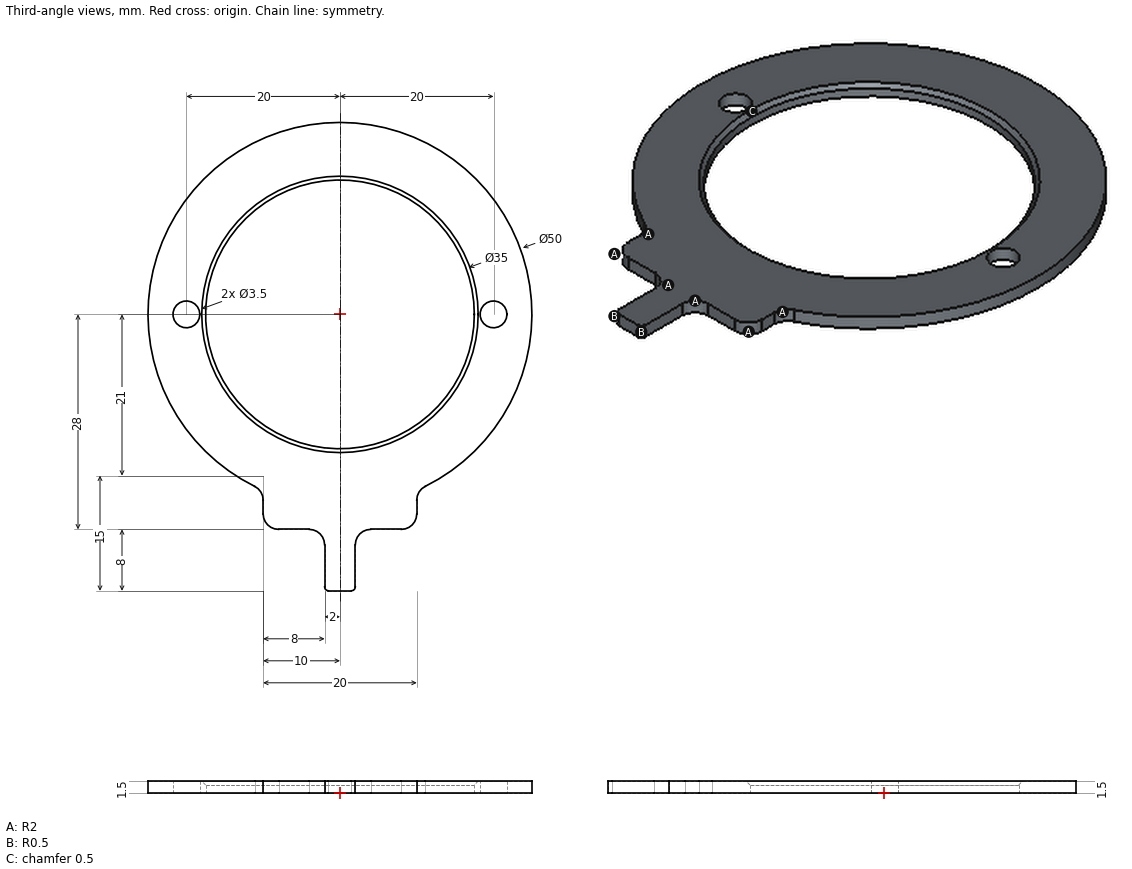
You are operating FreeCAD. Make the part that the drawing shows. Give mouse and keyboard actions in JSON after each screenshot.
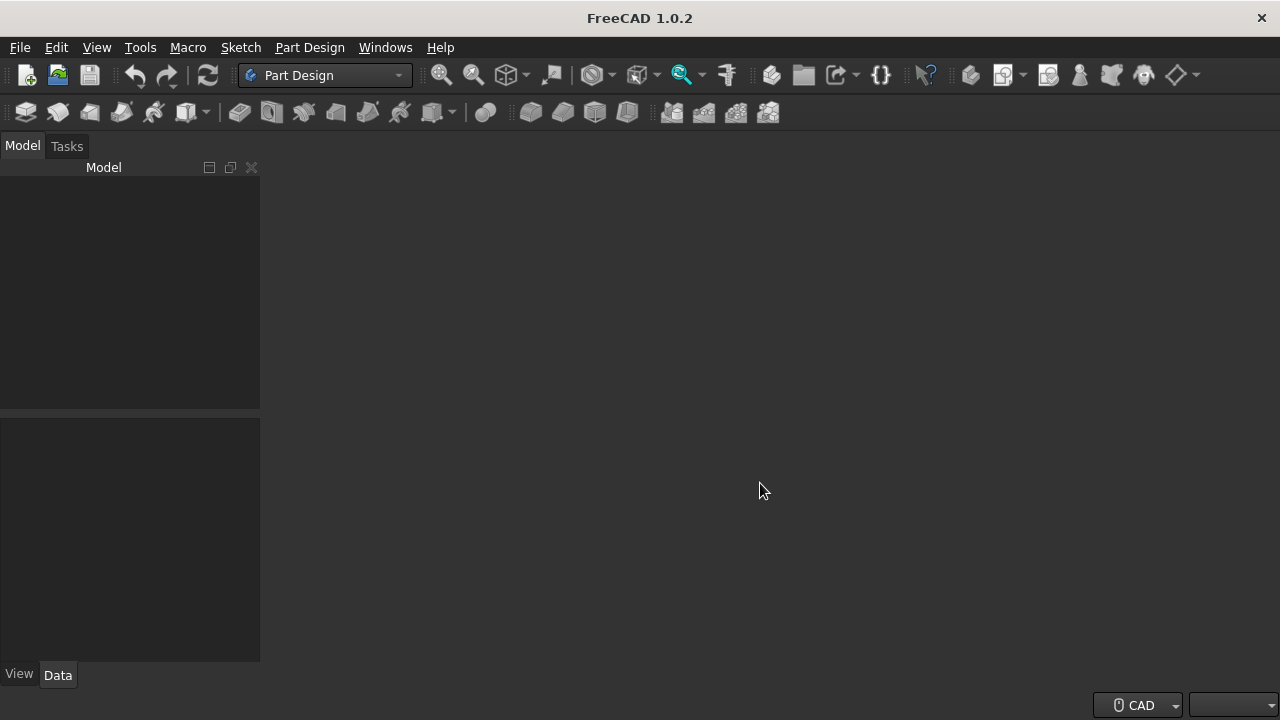
{"action": "left_click", "coordinate": [26, 76]}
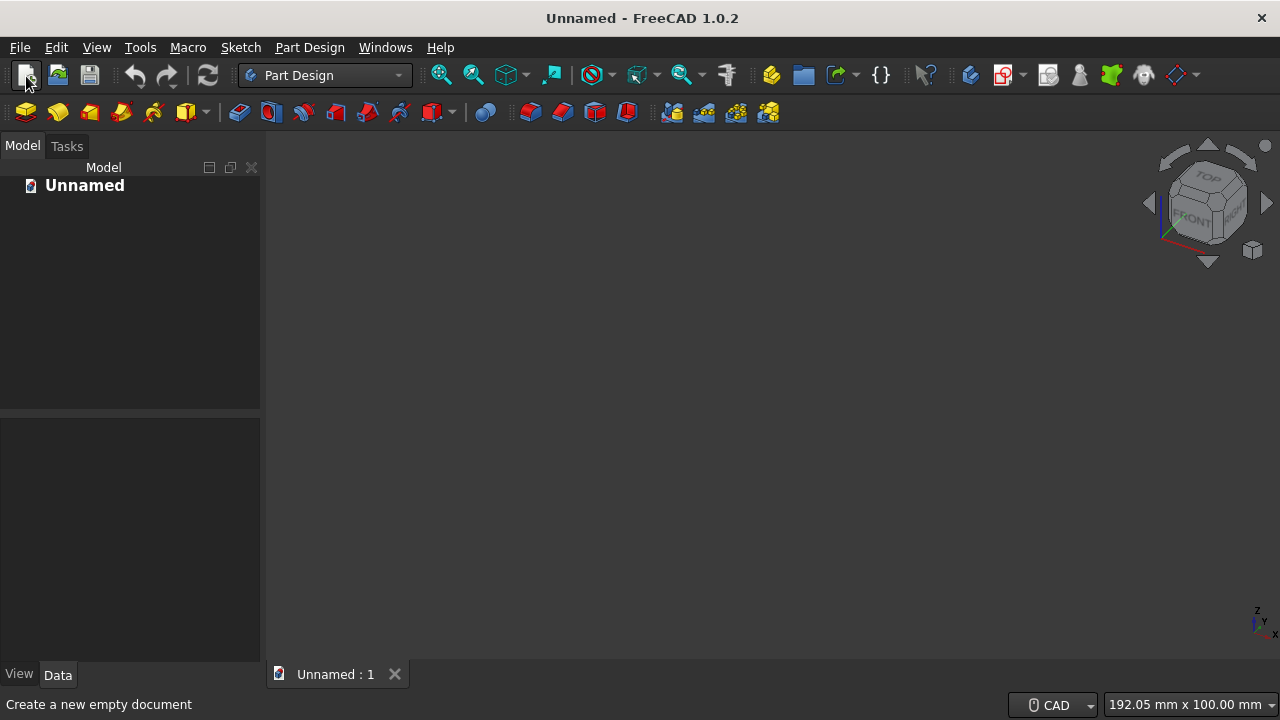
{"action": "left_click", "coordinate": [1004, 76]}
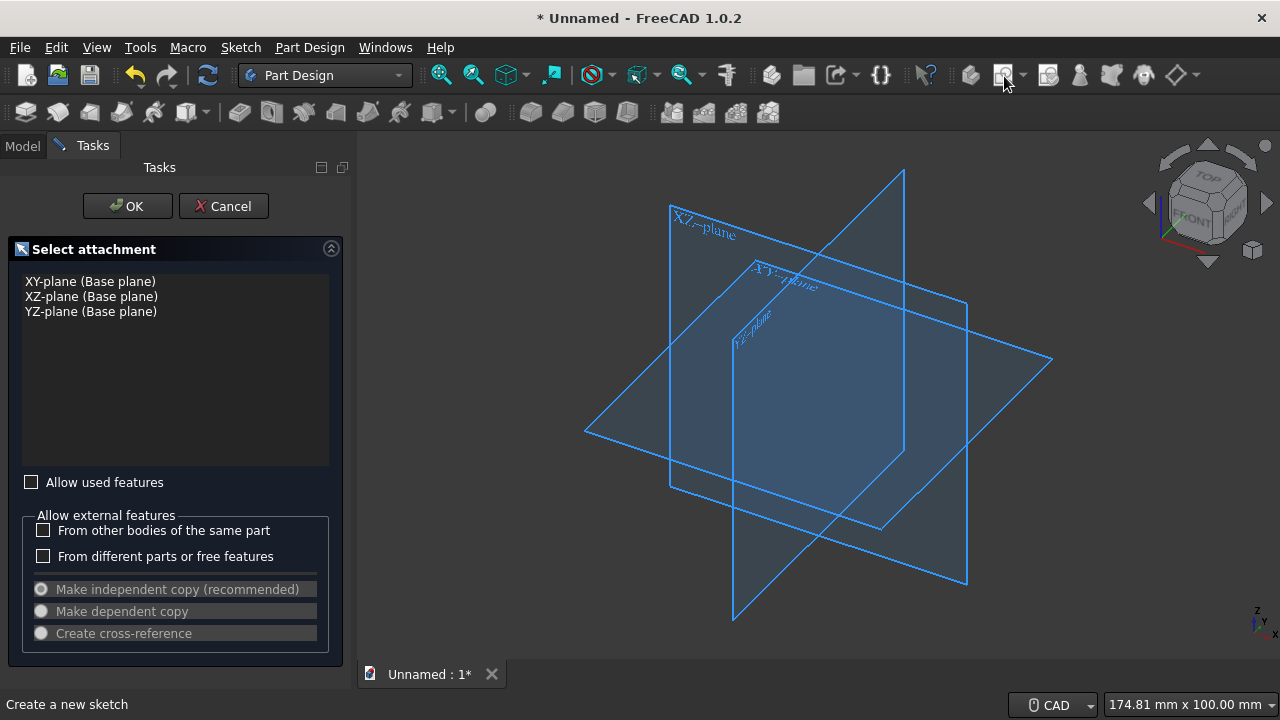
{"action": "left_click", "coordinate": [82, 282]}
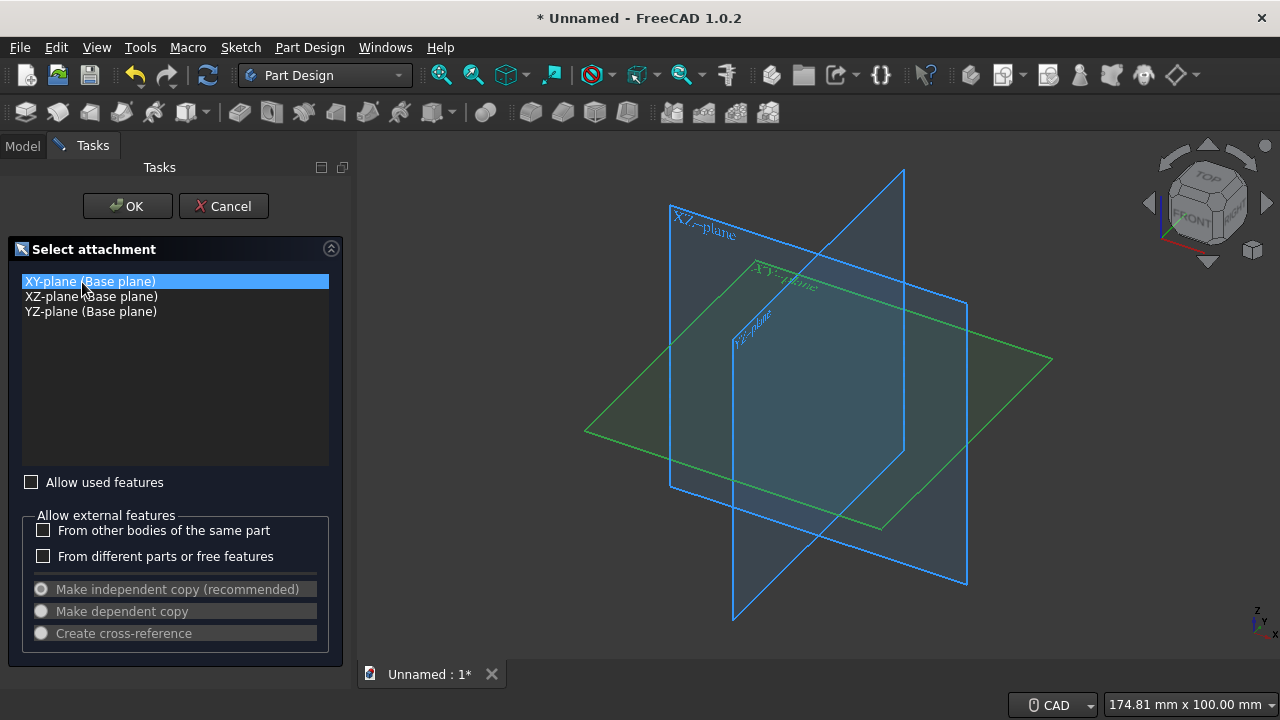
{"action": "left_click", "coordinate": [128, 206]}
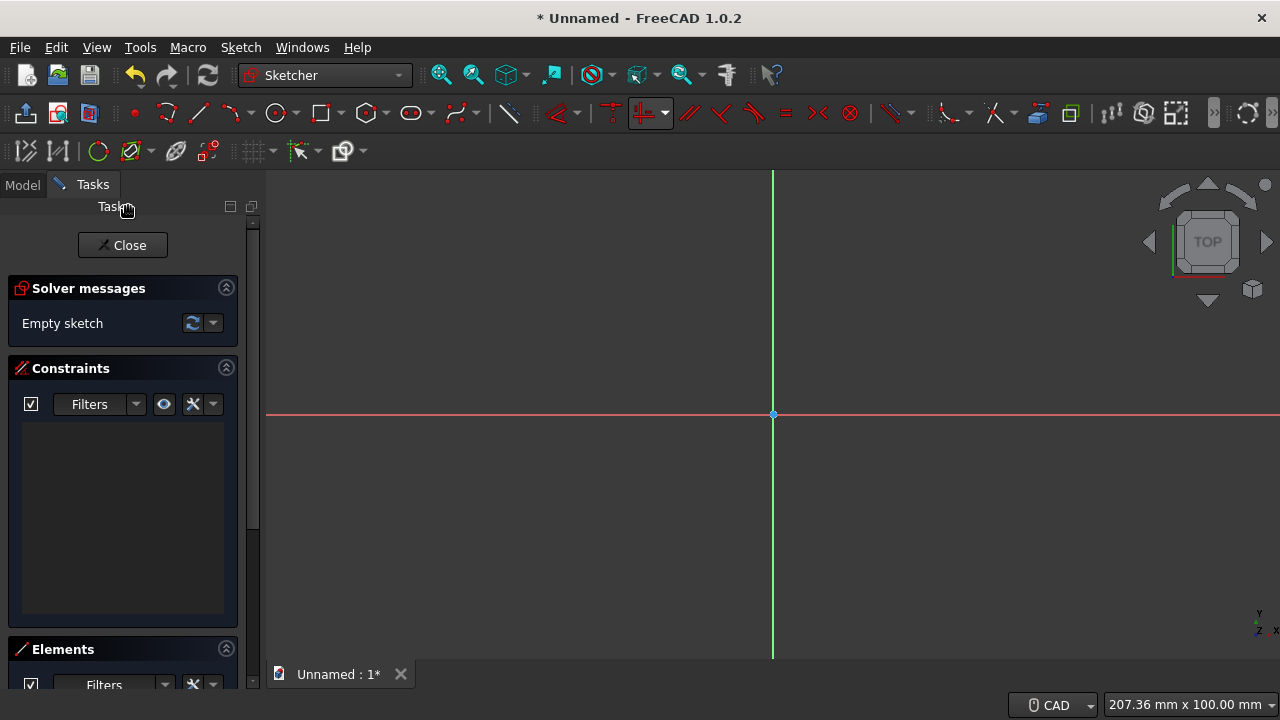
{"action": "left_click", "coordinate": [276, 114]}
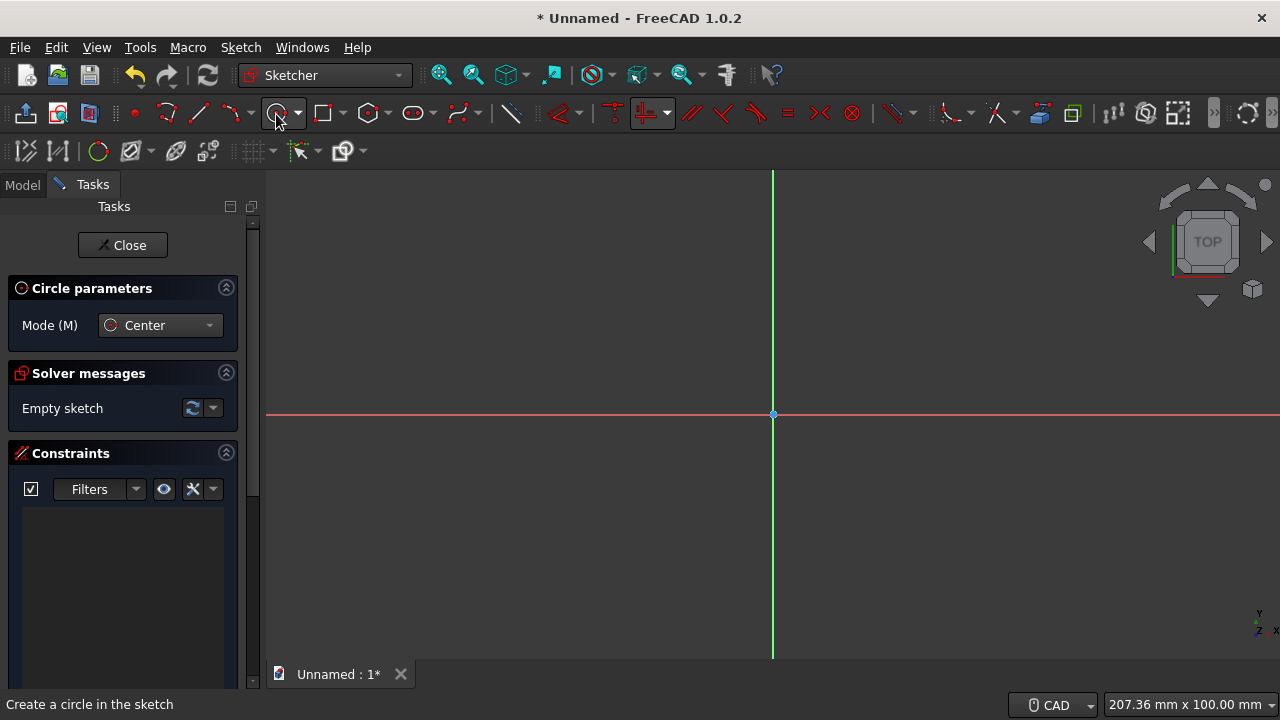
{"action": "left_click", "coordinate": [773, 414]}
{"action": "left_click", "coordinate": [859, 328]}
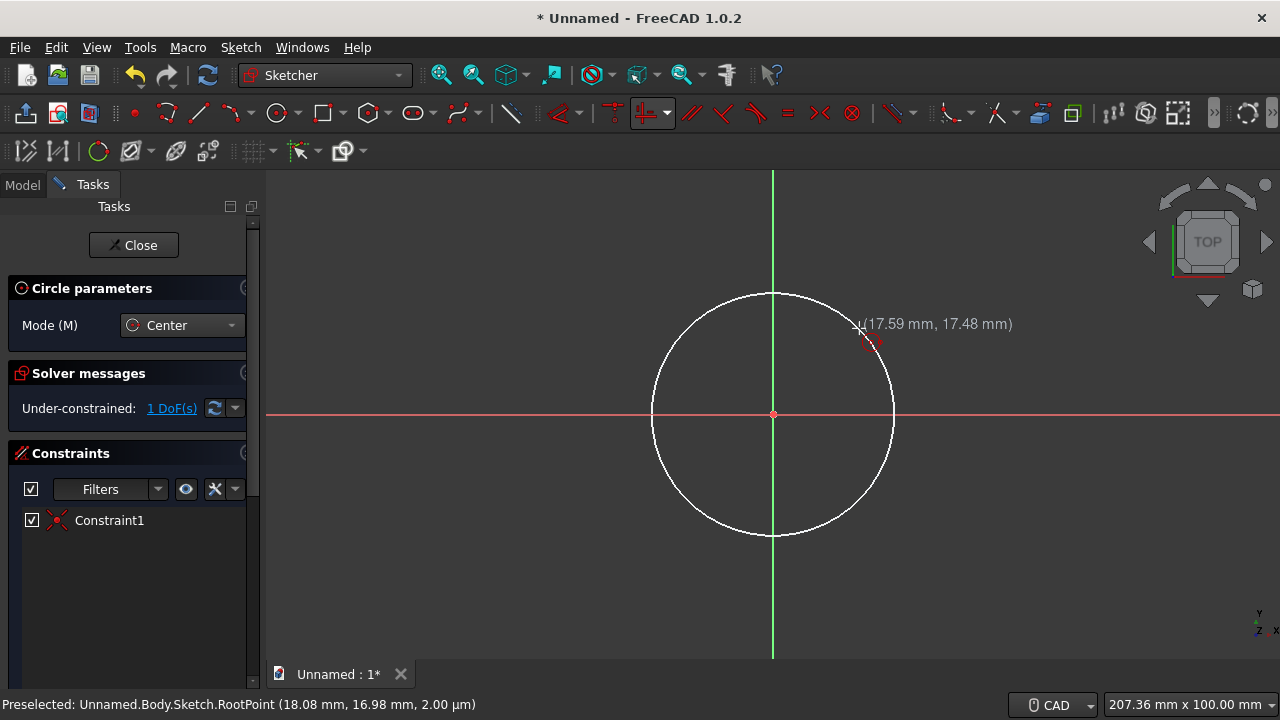
{"action": "left_click", "coordinate": [773, 414]}
{"action": "left_click", "coordinate": [834, 354]}
{"action": "key", "text": "Escape"}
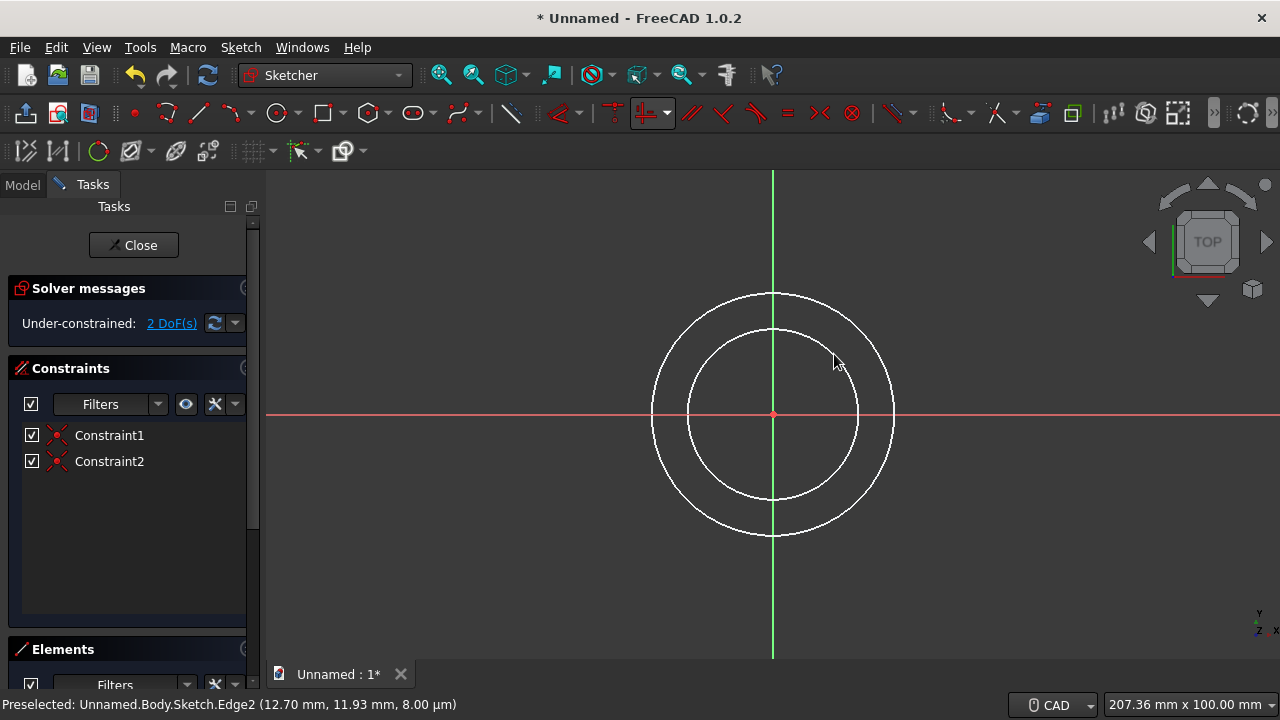
{"action": "left_click", "coordinate": [858, 328]}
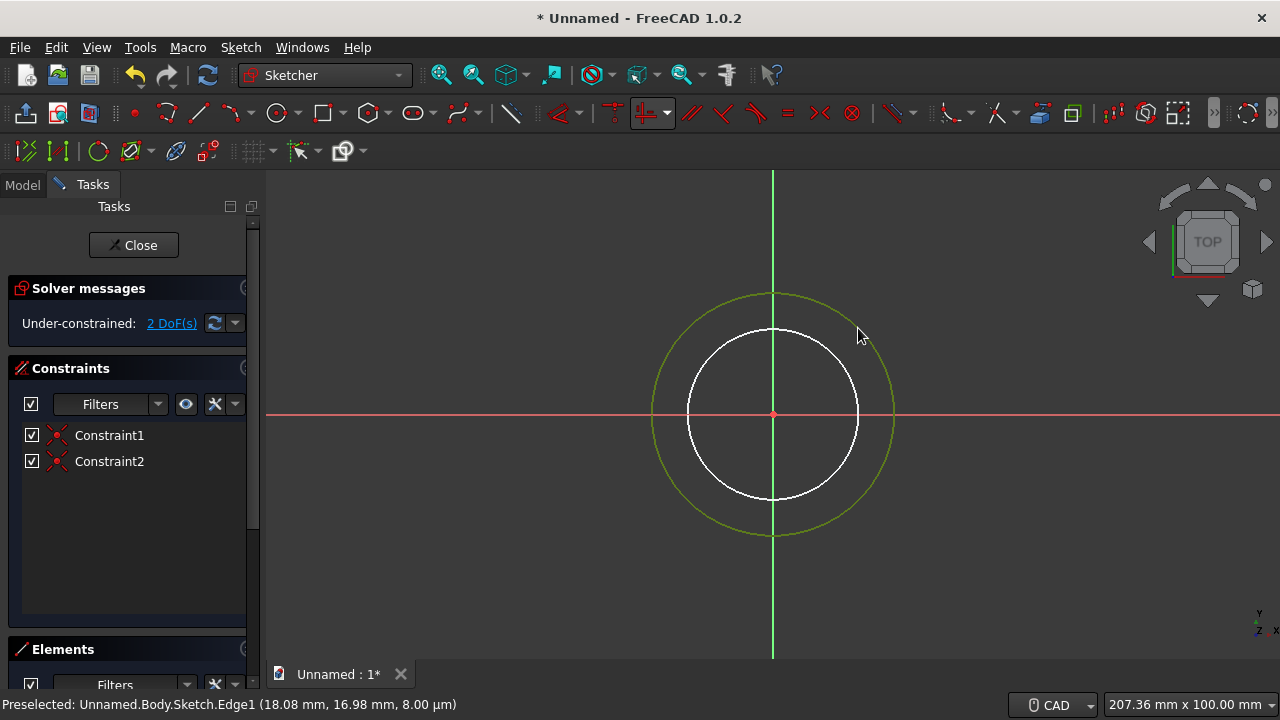
{"action": "left_click", "coordinate": [582, 114]}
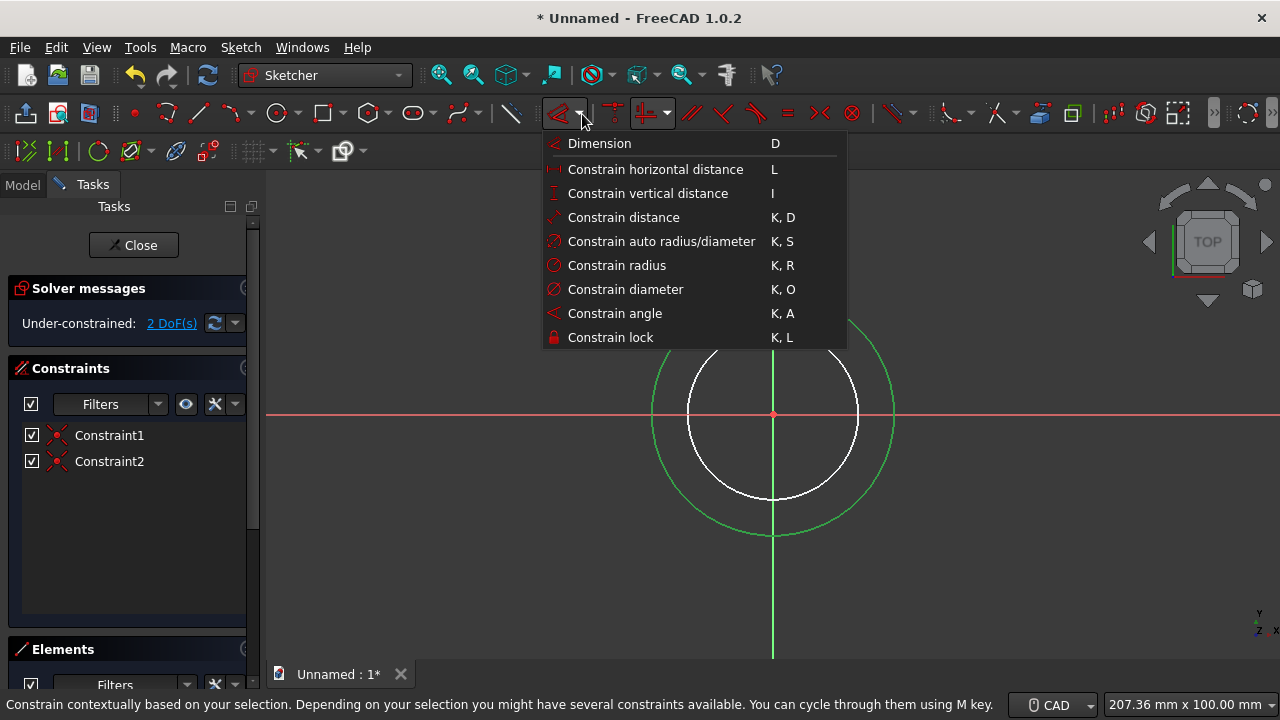
{"action": "left_click", "coordinate": [695, 289]}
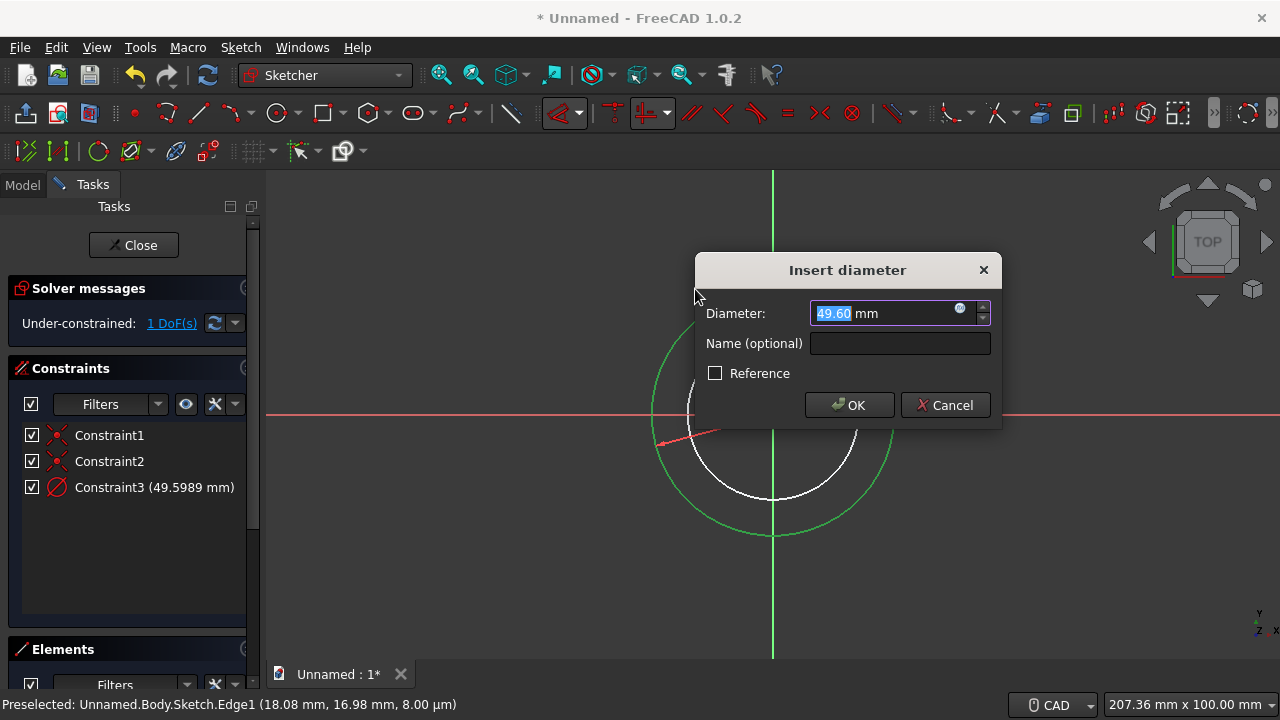
{"action": "type", "text": "50"}
{"action": "key", "text": "Return"}